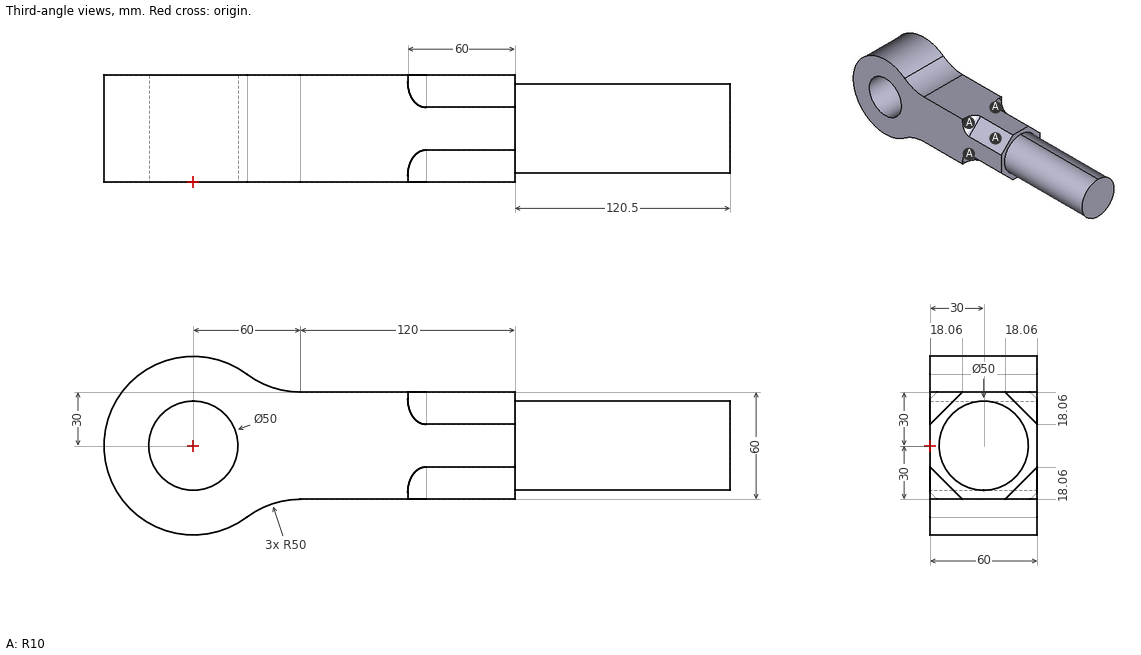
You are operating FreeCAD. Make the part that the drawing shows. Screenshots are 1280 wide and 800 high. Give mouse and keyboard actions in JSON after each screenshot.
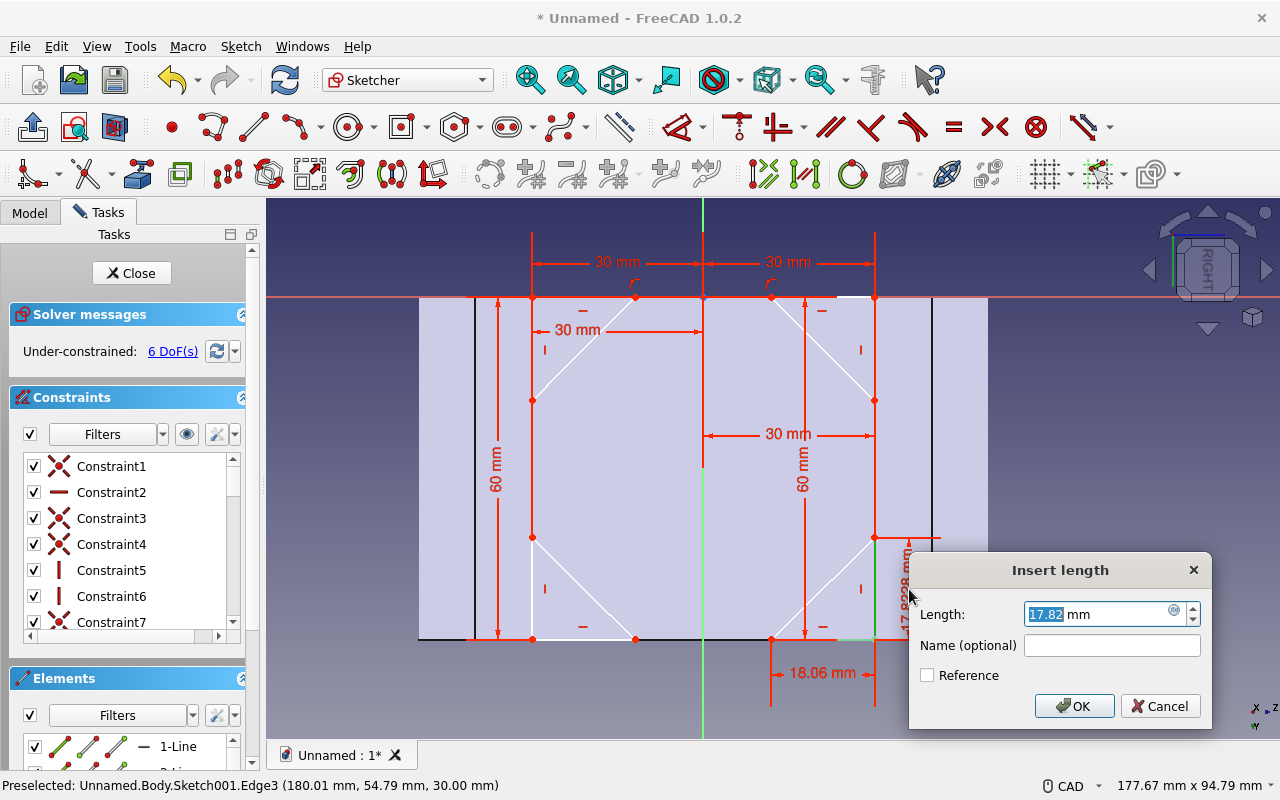
{"action": "type", "text": "18.06"}
{"action": "key", "text": "Return"}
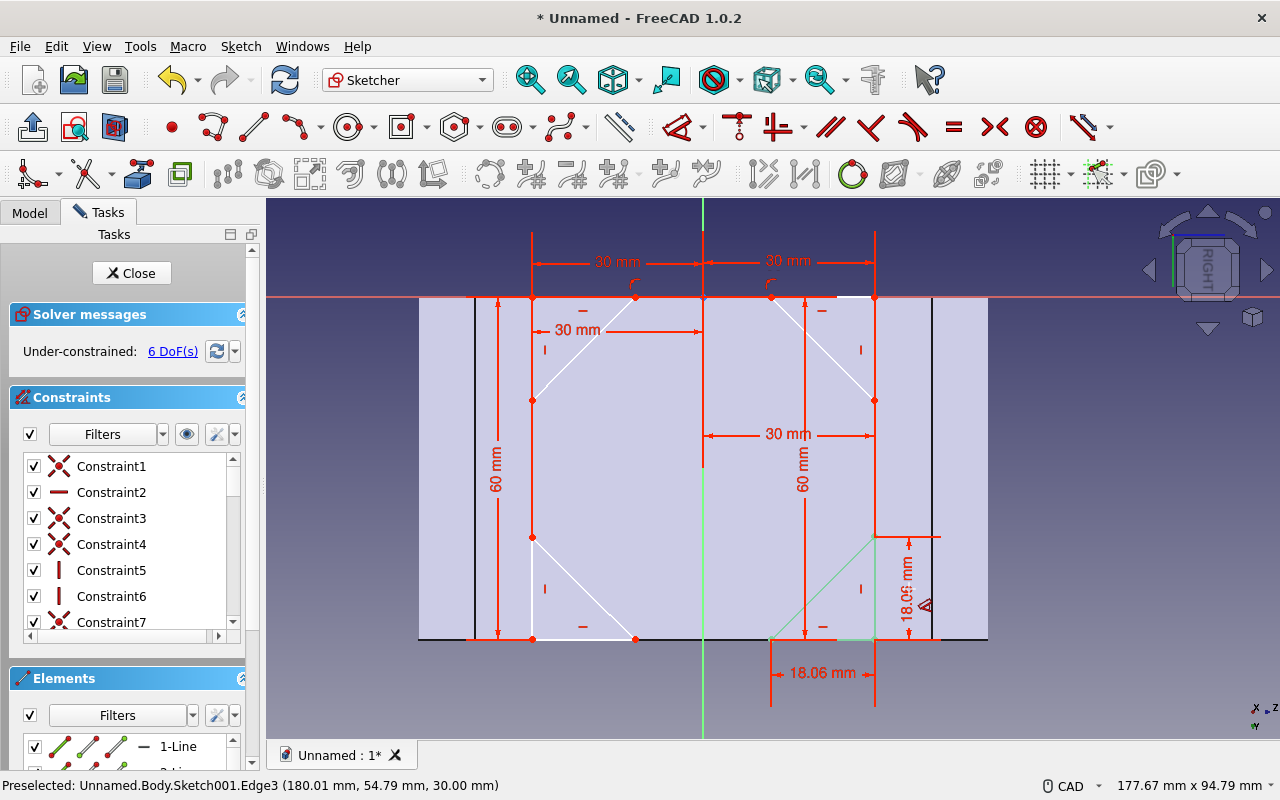
{"action": "left_click", "coordinate": [532, 569]}
{"action": "left_click", "coordinate": [498, 589]}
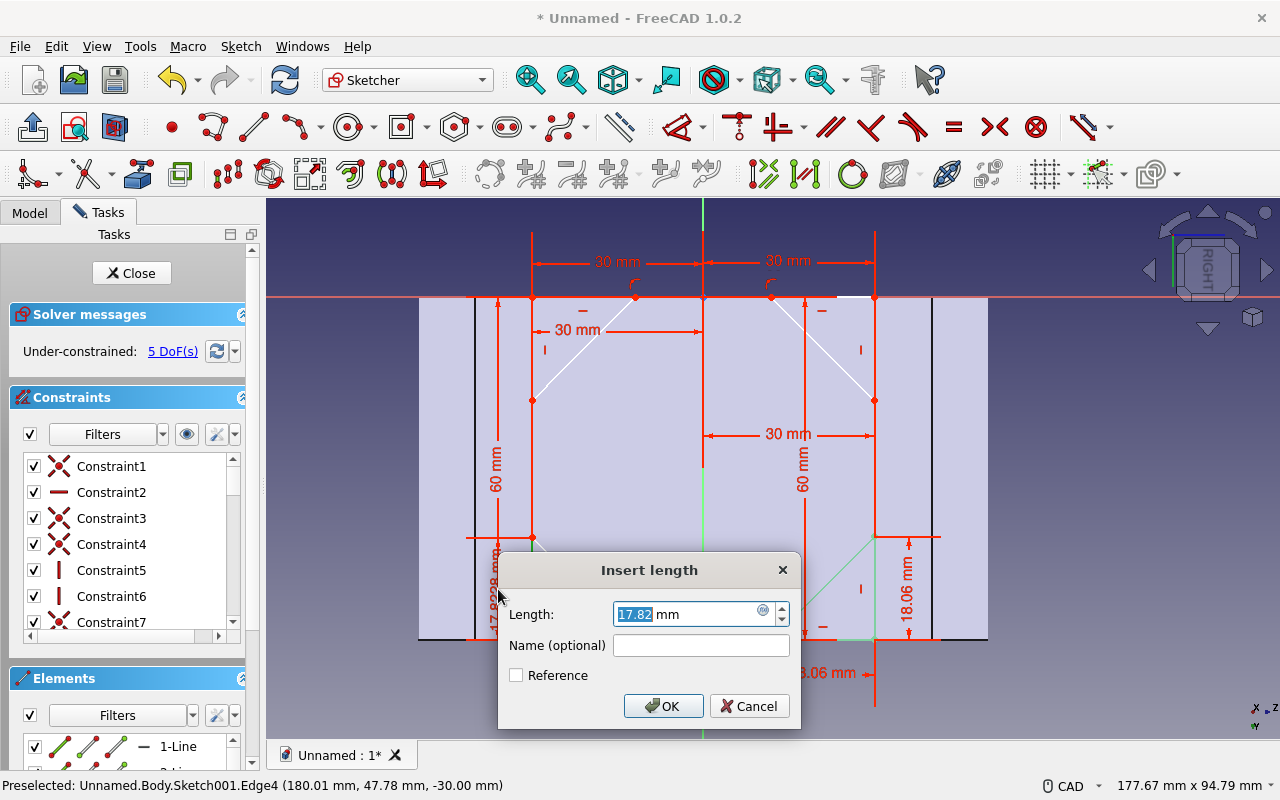
{"action": "type", "text": "18.06"}
{"action": "key", "text": "Return"}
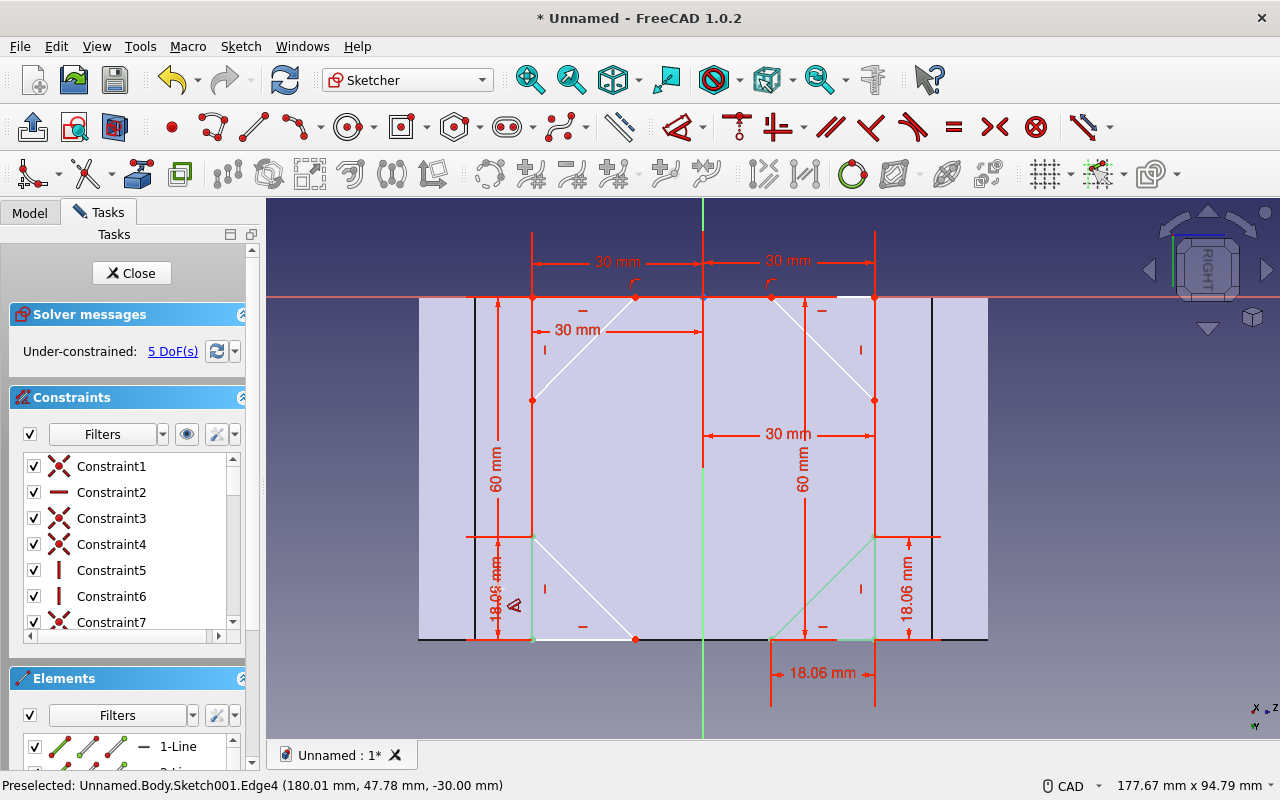
{"action": "left_click", "coordinate": [563, 640]}
{"action": "left_click", "coordinate": [584, 674]}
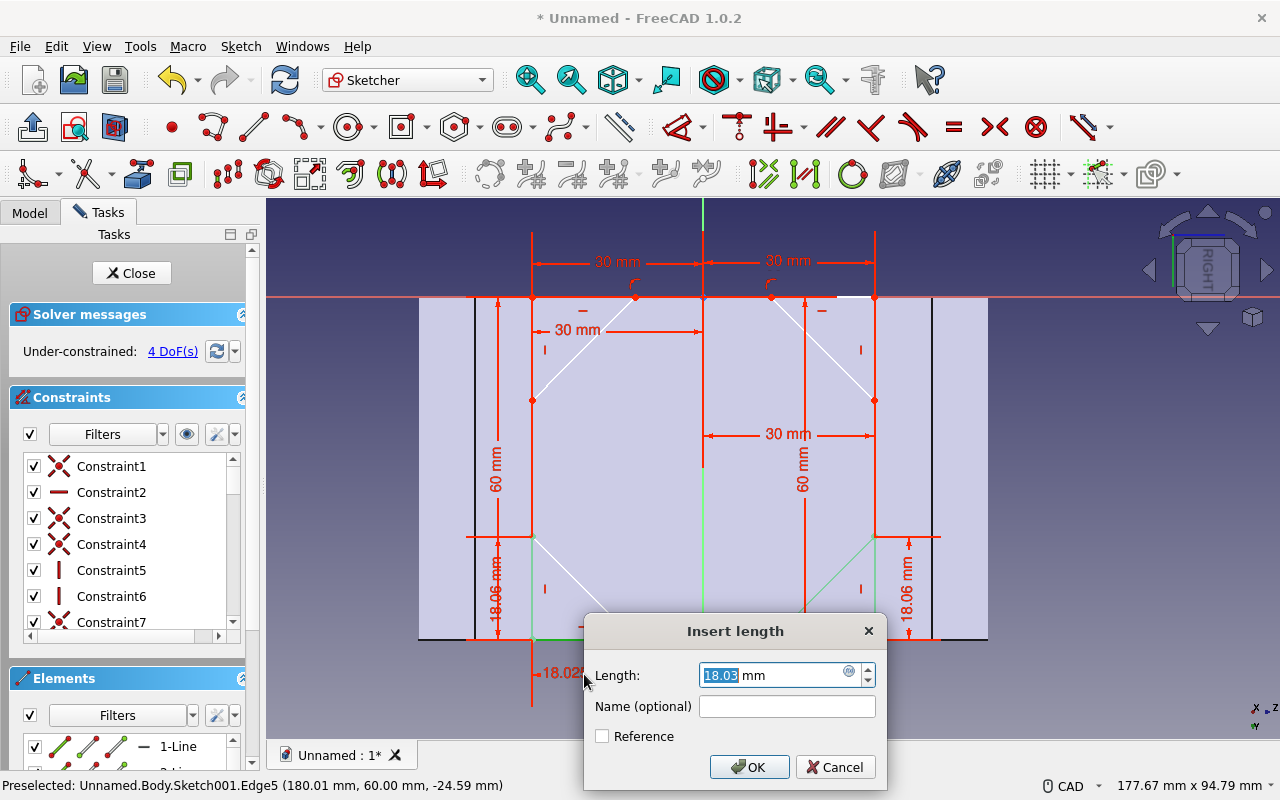
{"action": "type", "text": "18.06"}
{"action": "key", "text": "Return"}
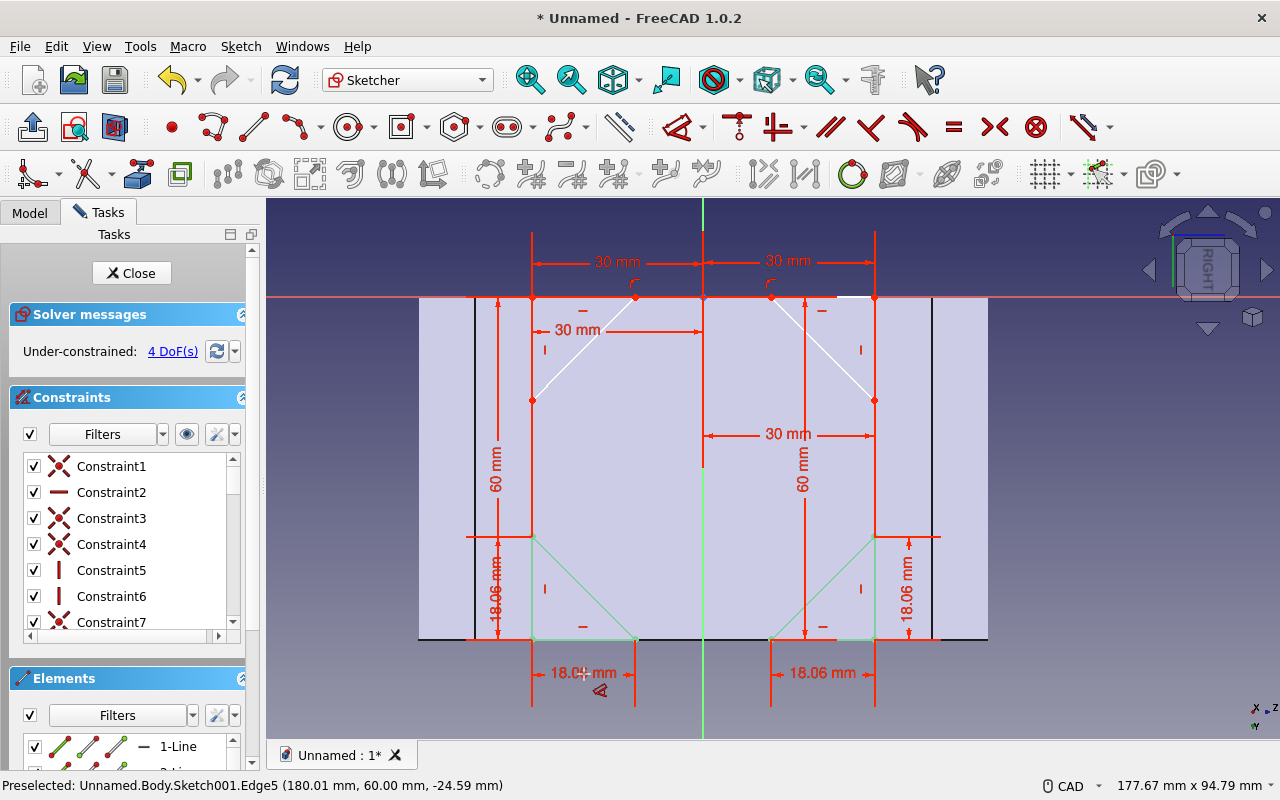
{"action": "left_click", "coordinate": [875, 370]}
{"action": "left_click", "coordinate": [909, 349]}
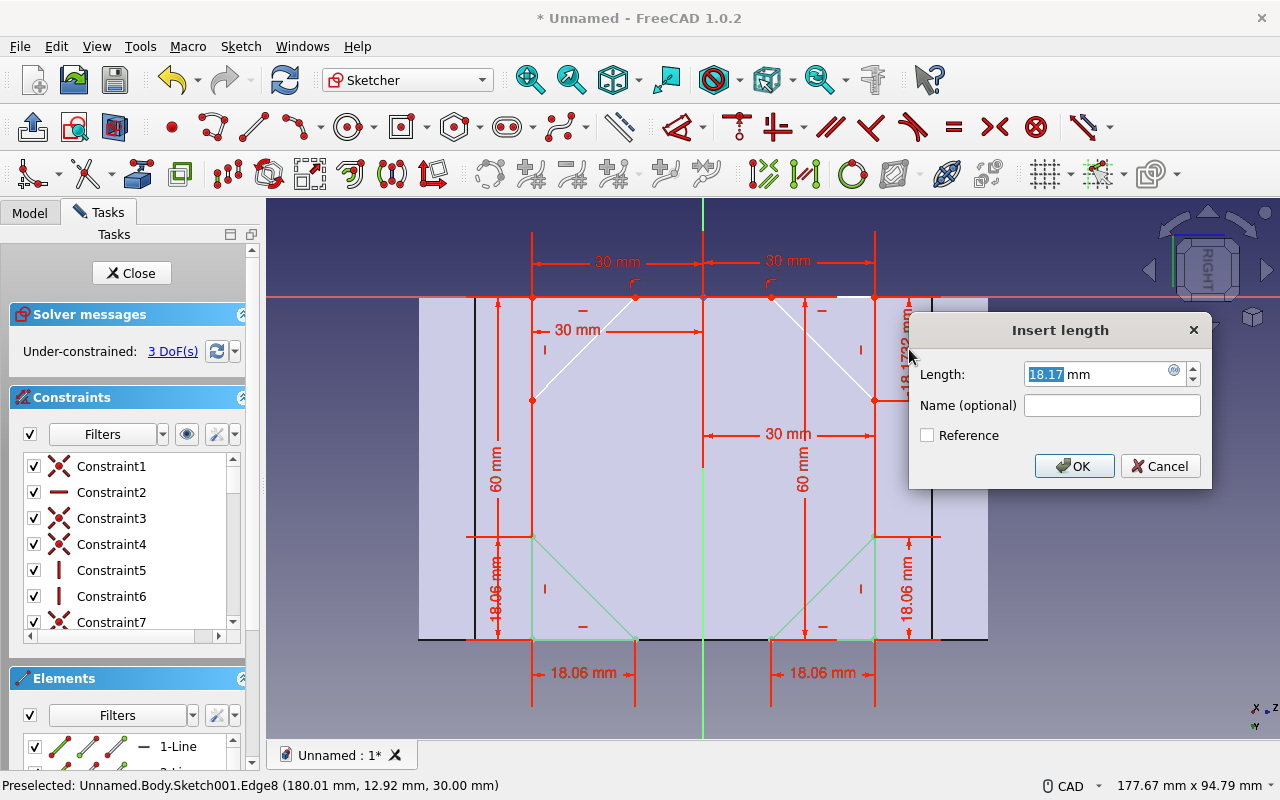
{"action": "type", "text": "18.06"}
{"action": "key", "text": "Return"}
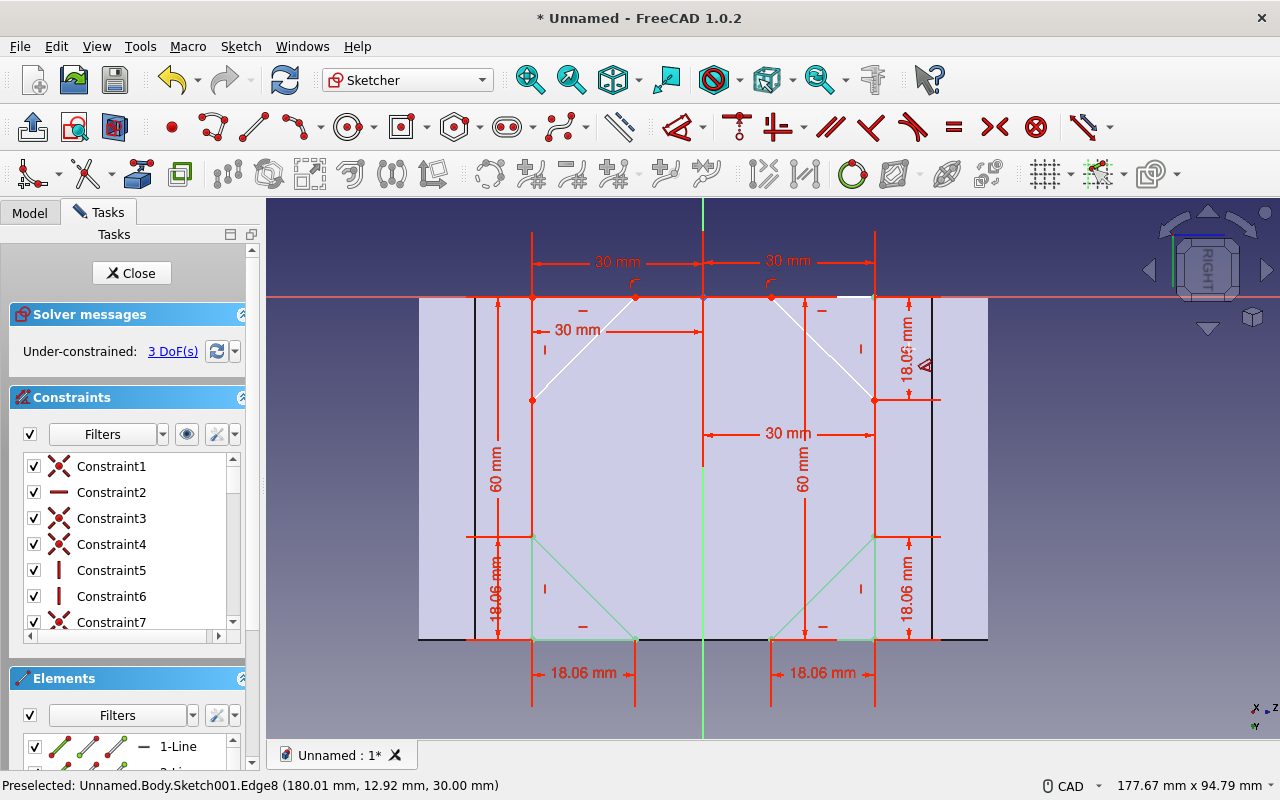
{"action": "left_click", "coordinate": [843, 297]}
{"action": "left_click", "coordinate": [787, 331]}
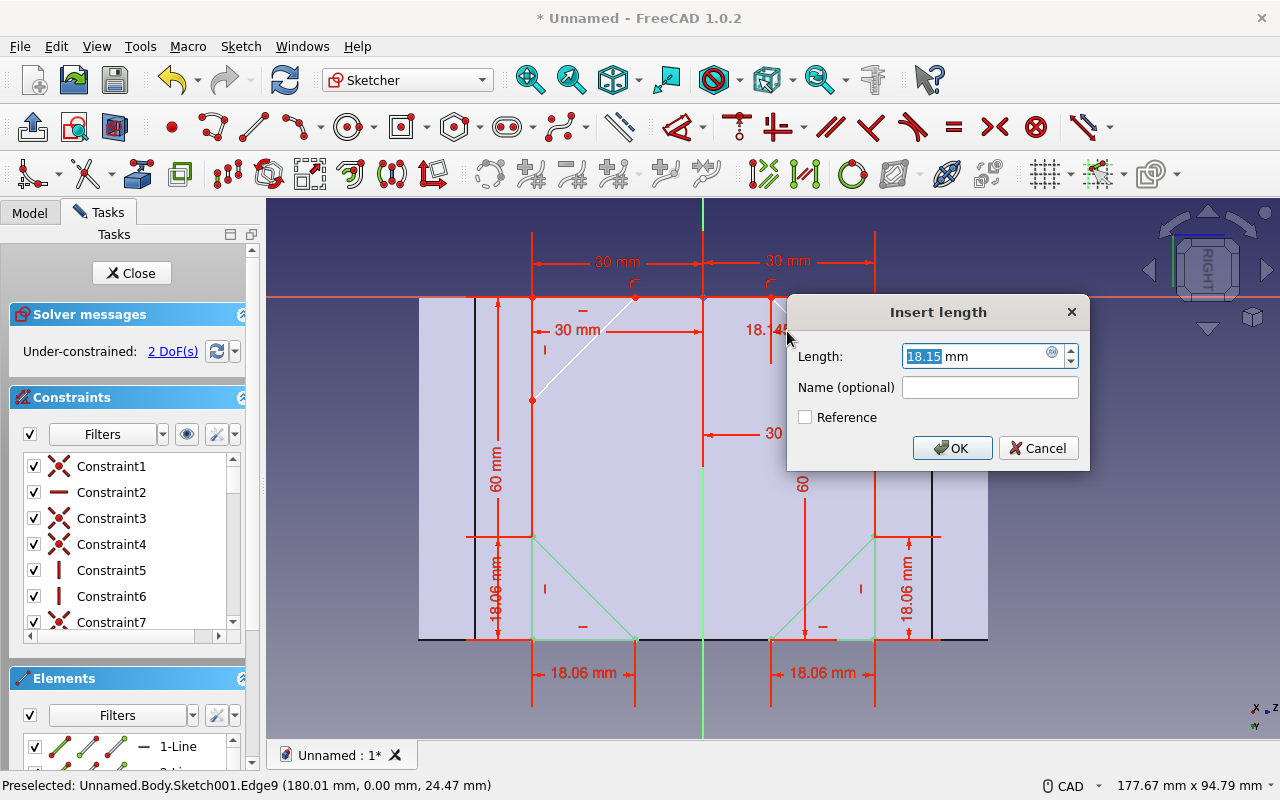
{"action": "type", "text": "18.06"}
{"action": "key", "text": "Return"}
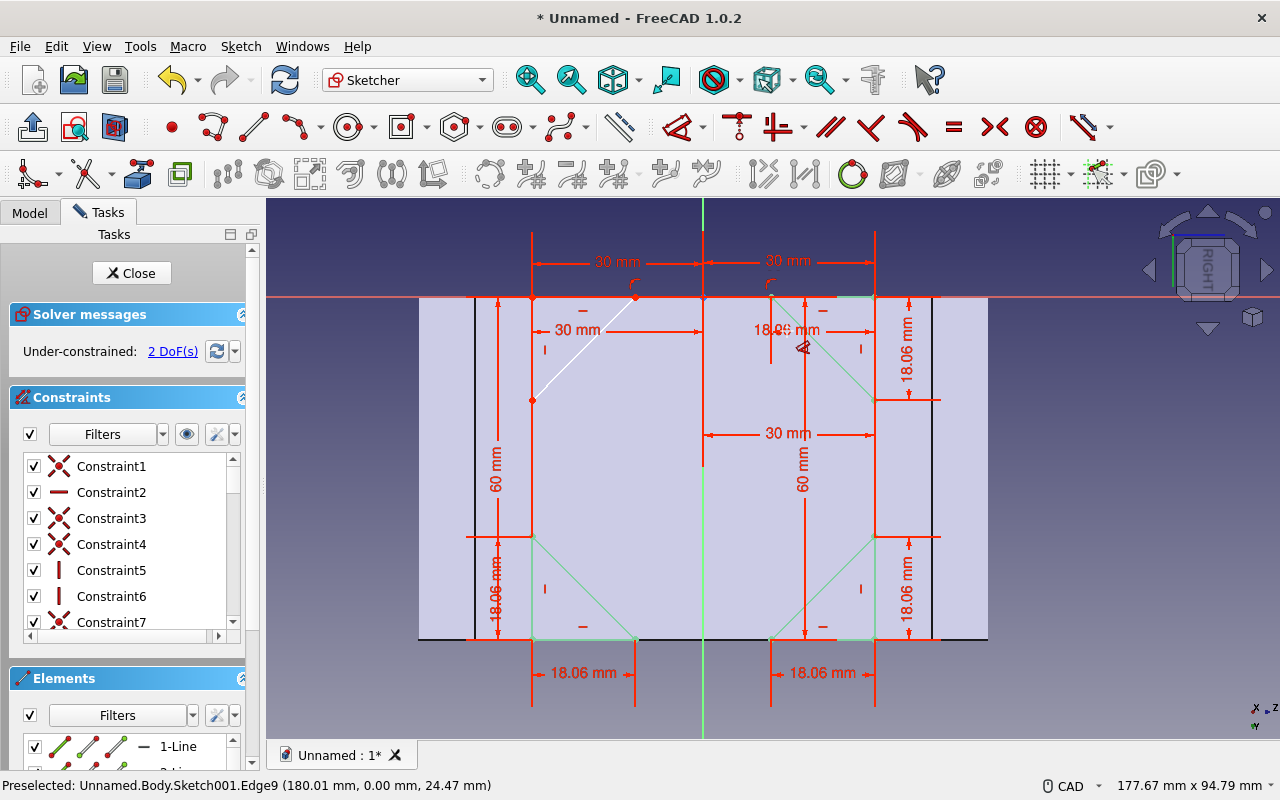
{"action": "left_click", "coordinate": [604, 297]}
{"action": "left_click", "coordinate": [548, 263]}